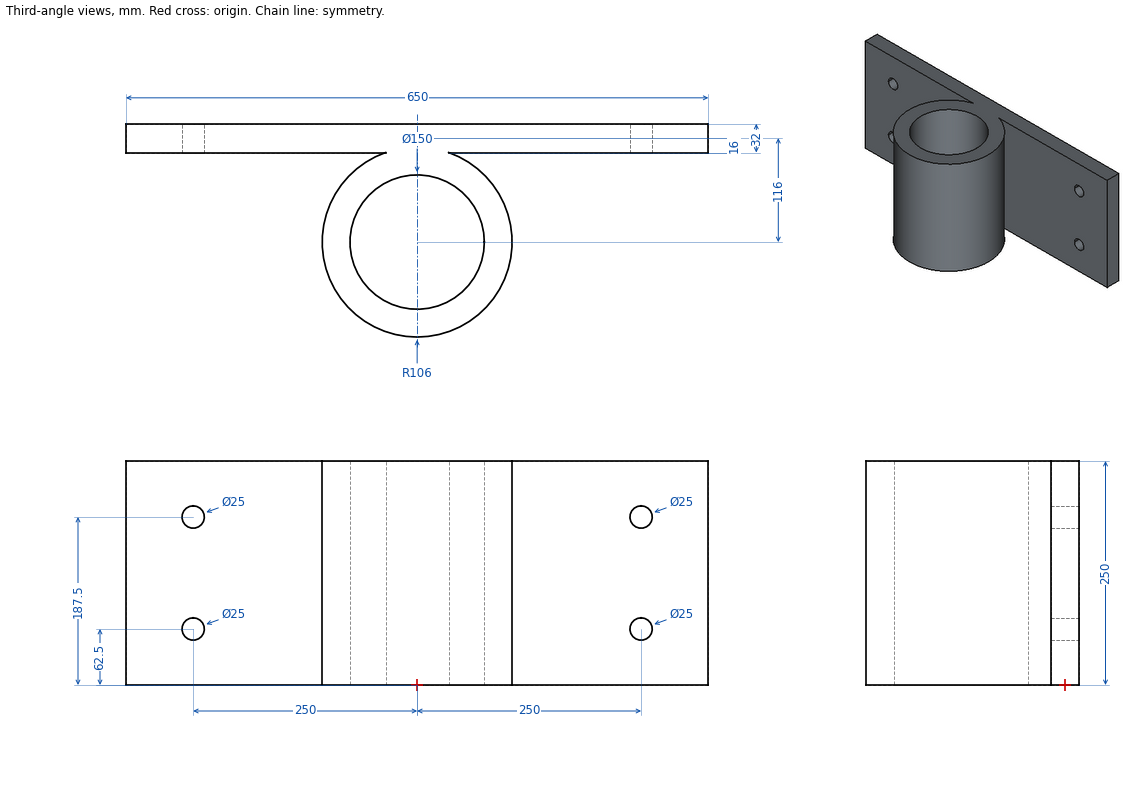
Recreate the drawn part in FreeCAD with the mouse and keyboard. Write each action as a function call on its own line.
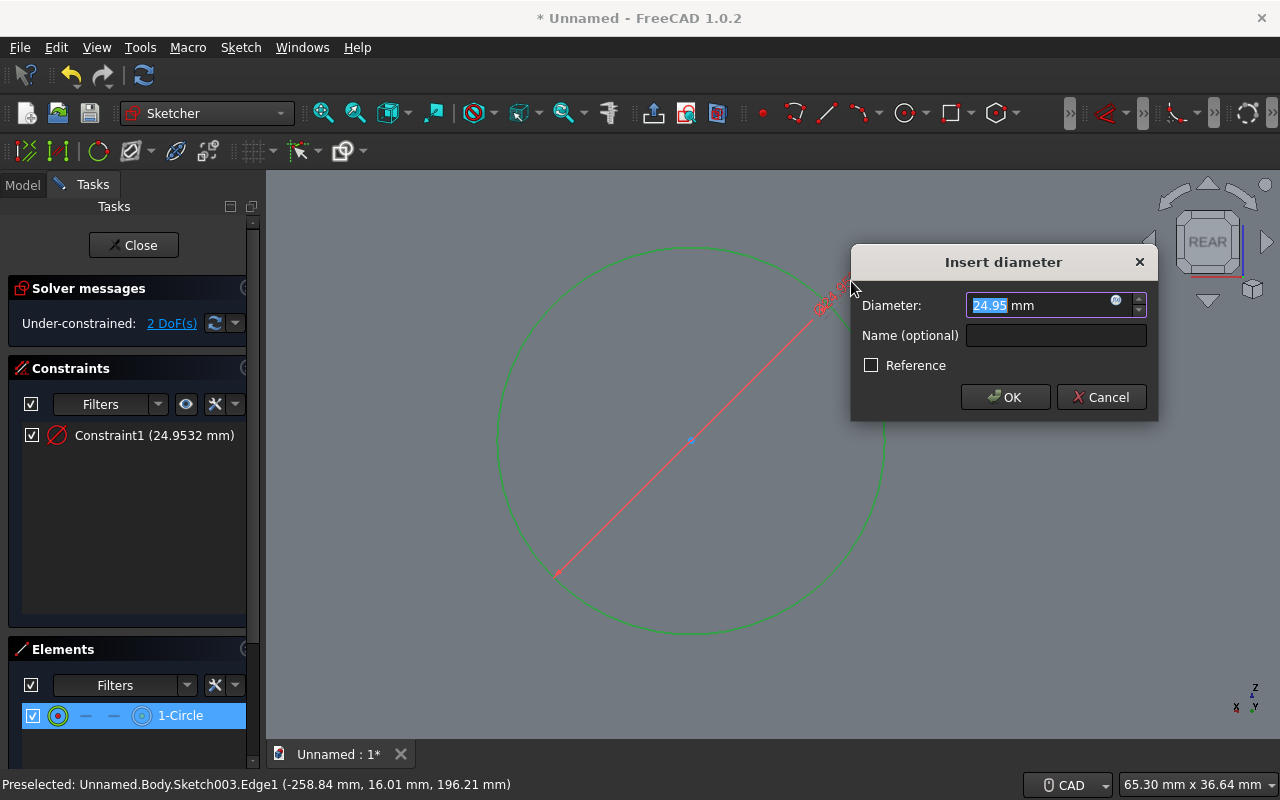
text(25)
key(Return)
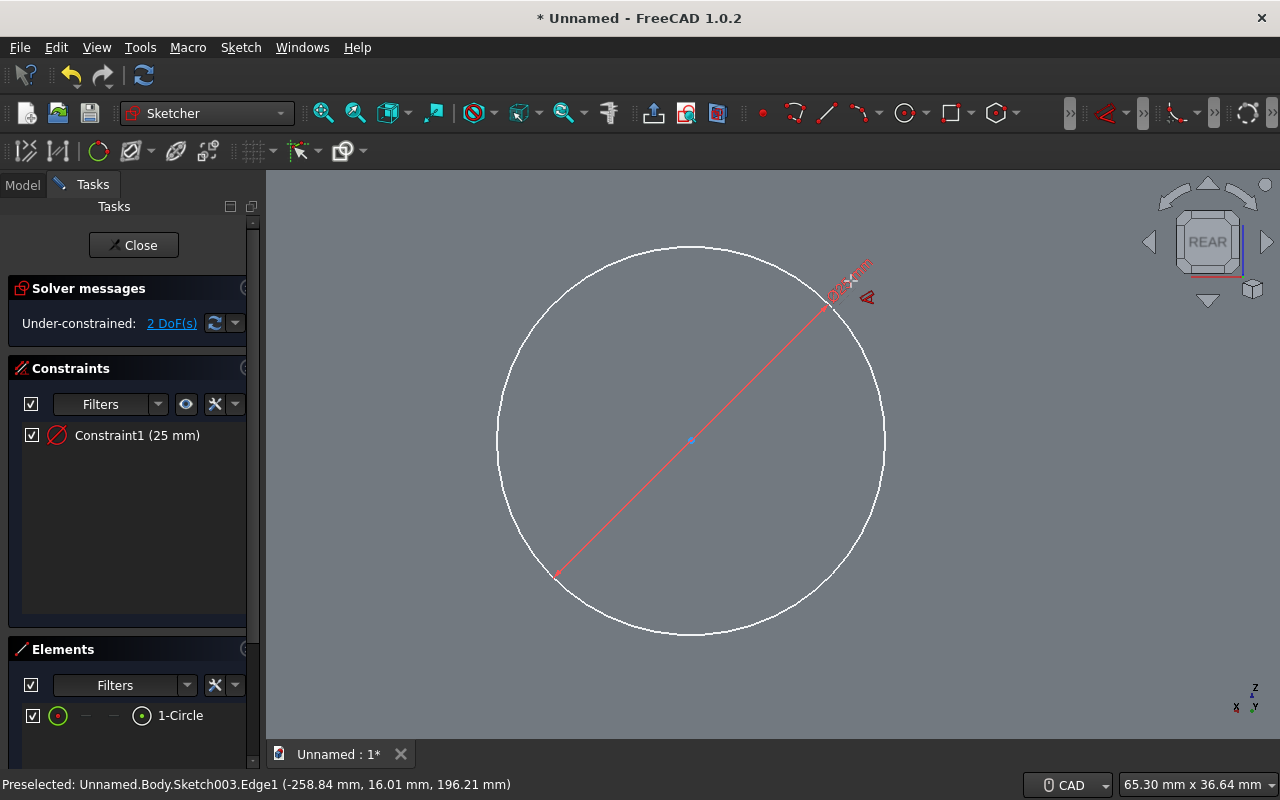
click(691, 441)
click(401, 407)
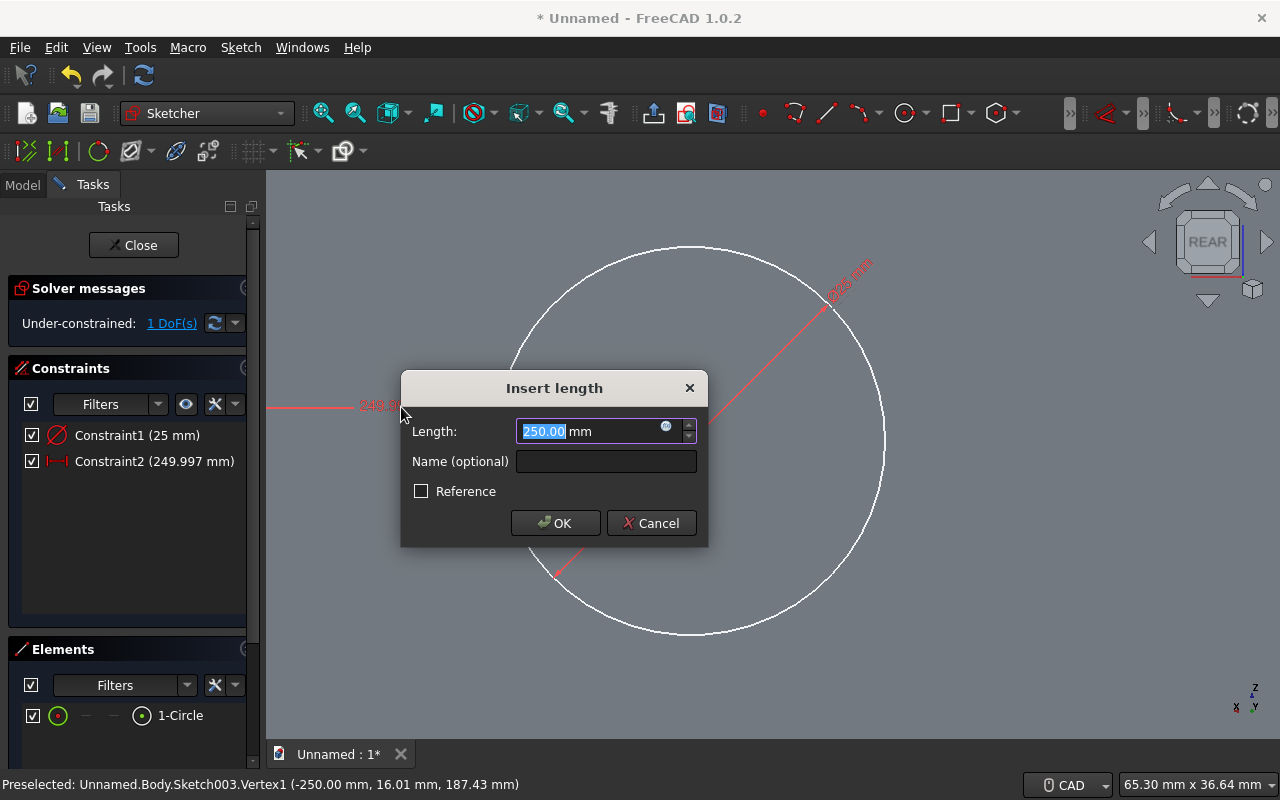
text(250)
key(Return)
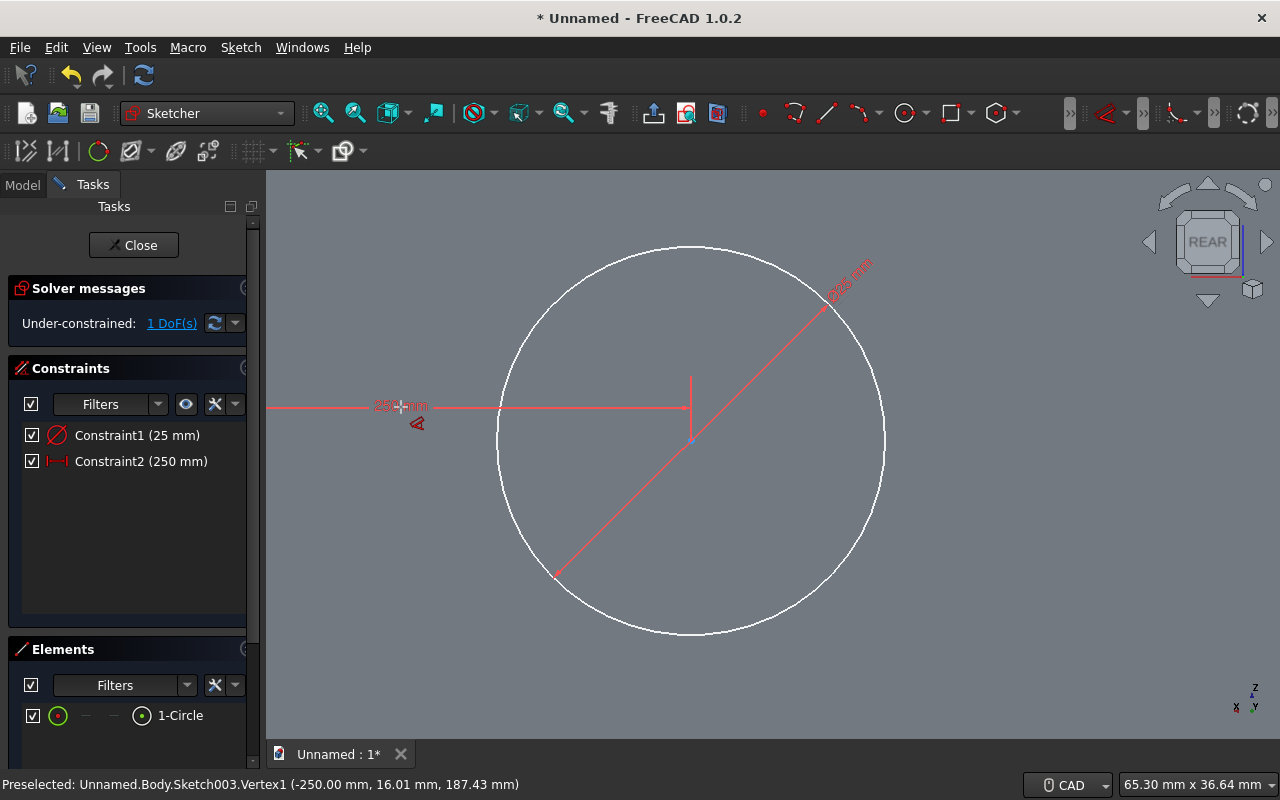
click(691, 441)
click(725, 576)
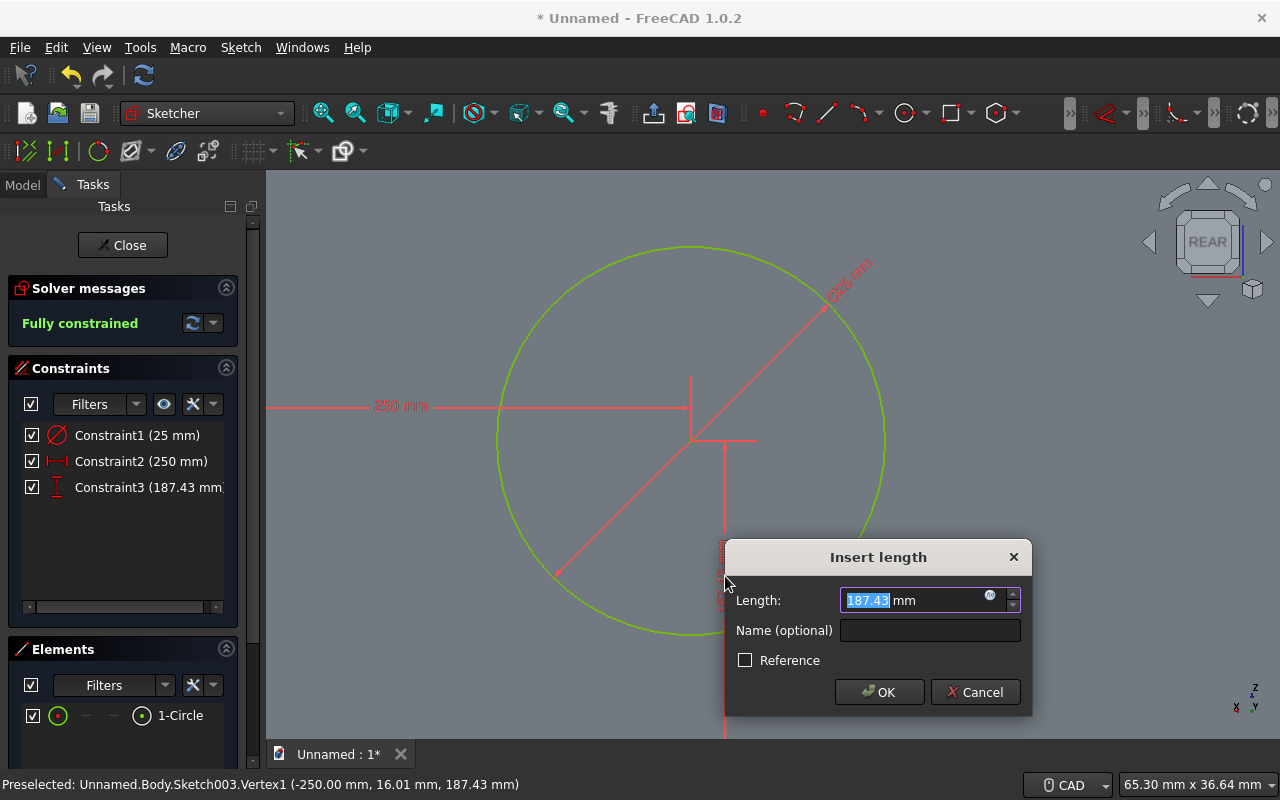
text(187.5)
key(Return)
key(Escape)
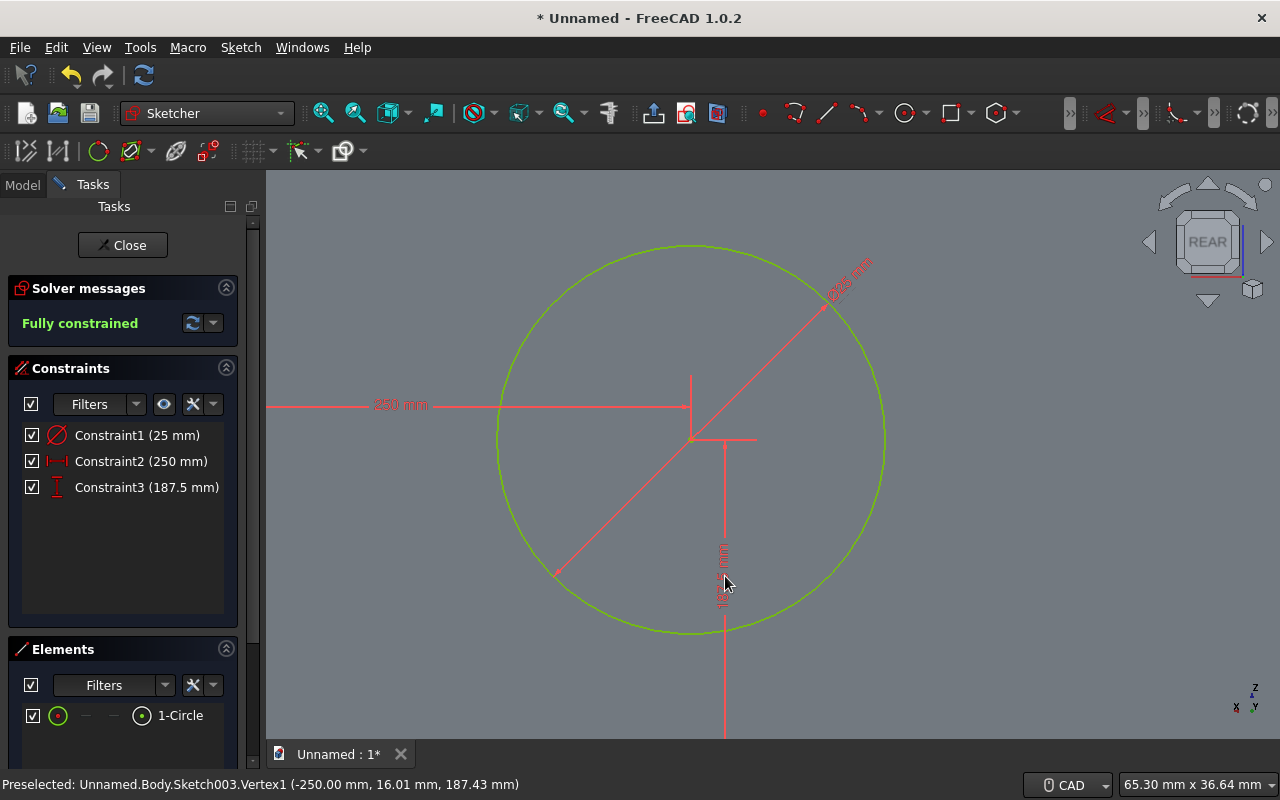
click(123, 245)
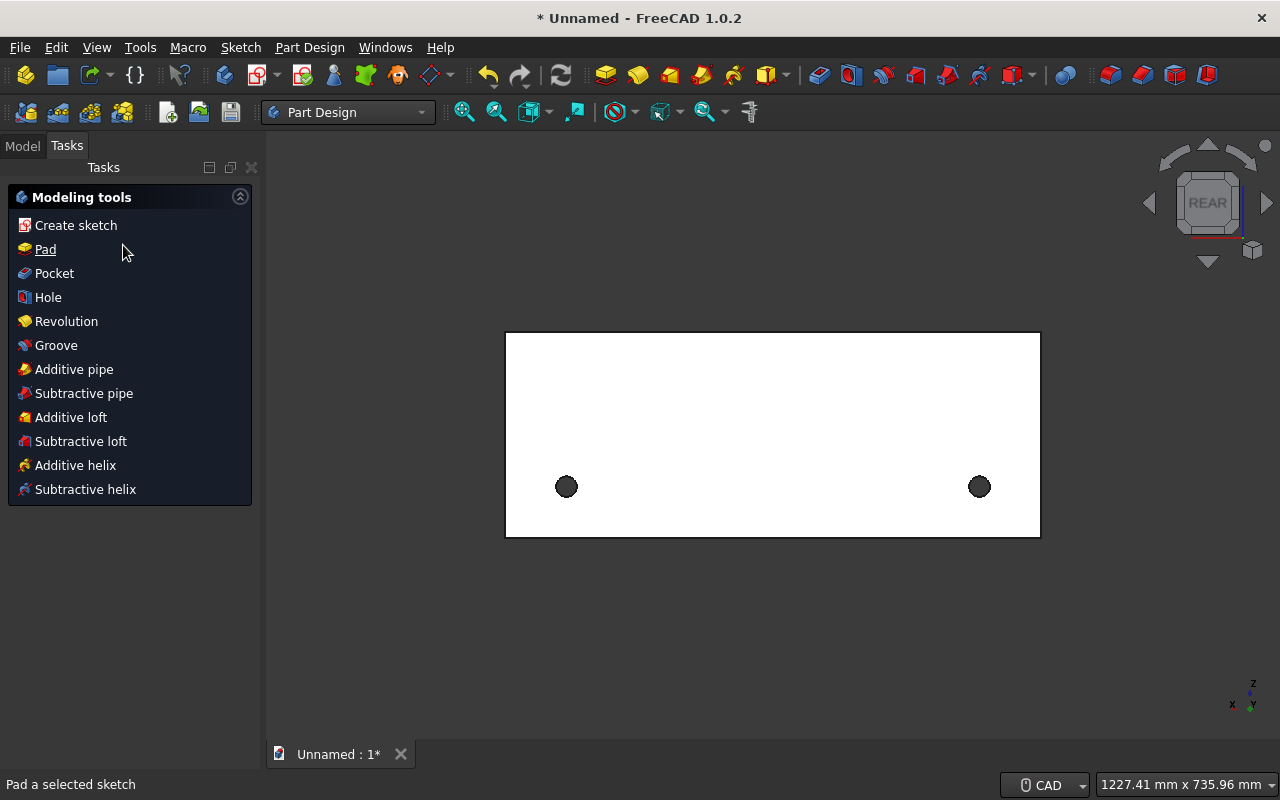
click(820, 76)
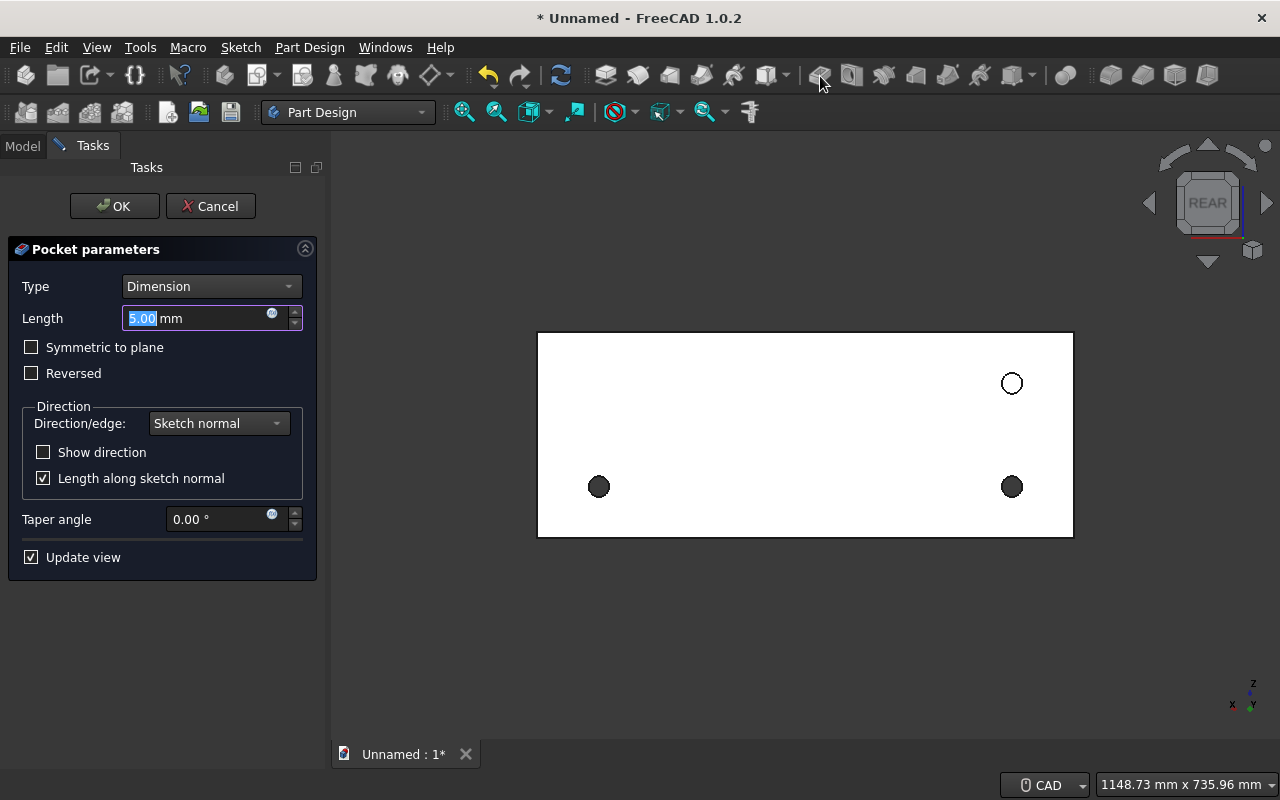
click(212, 286)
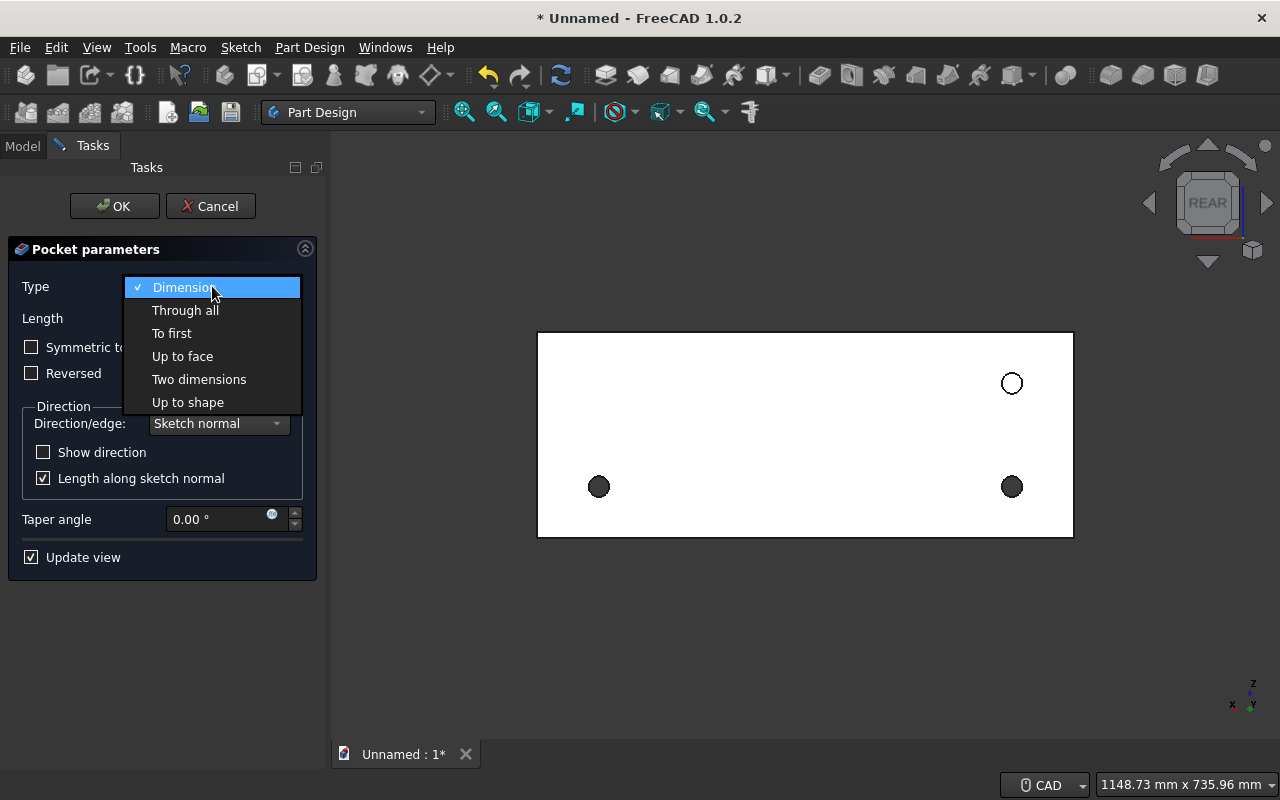
click(212, 334)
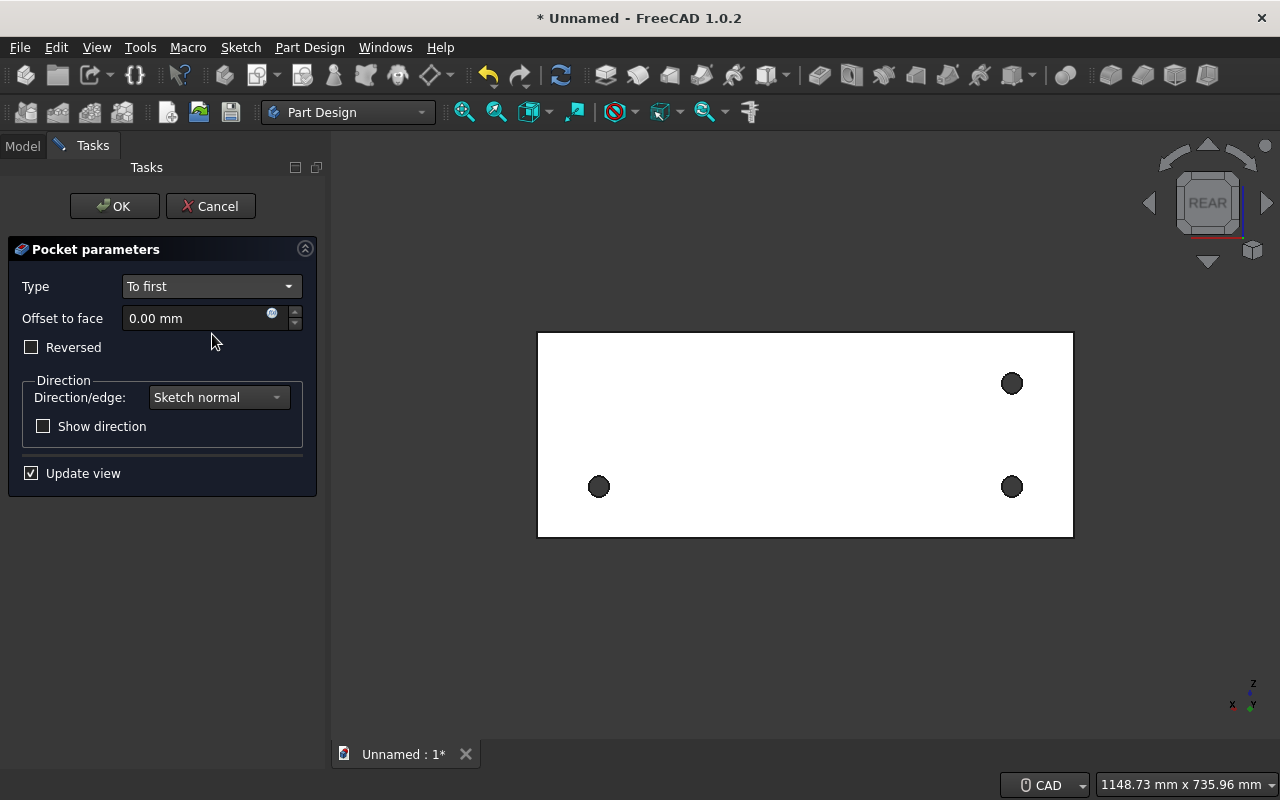
click(115, 206)